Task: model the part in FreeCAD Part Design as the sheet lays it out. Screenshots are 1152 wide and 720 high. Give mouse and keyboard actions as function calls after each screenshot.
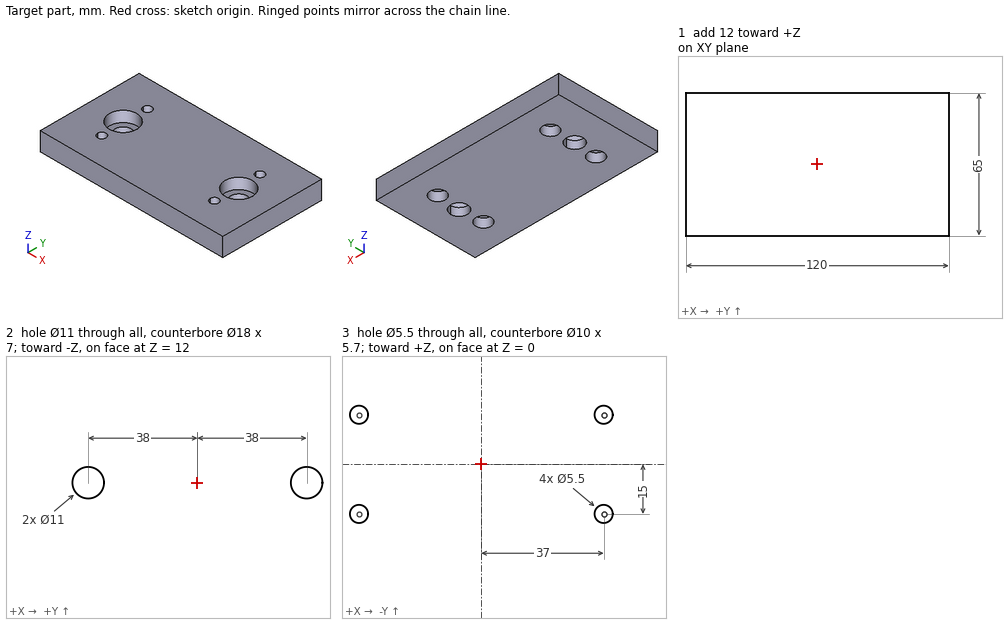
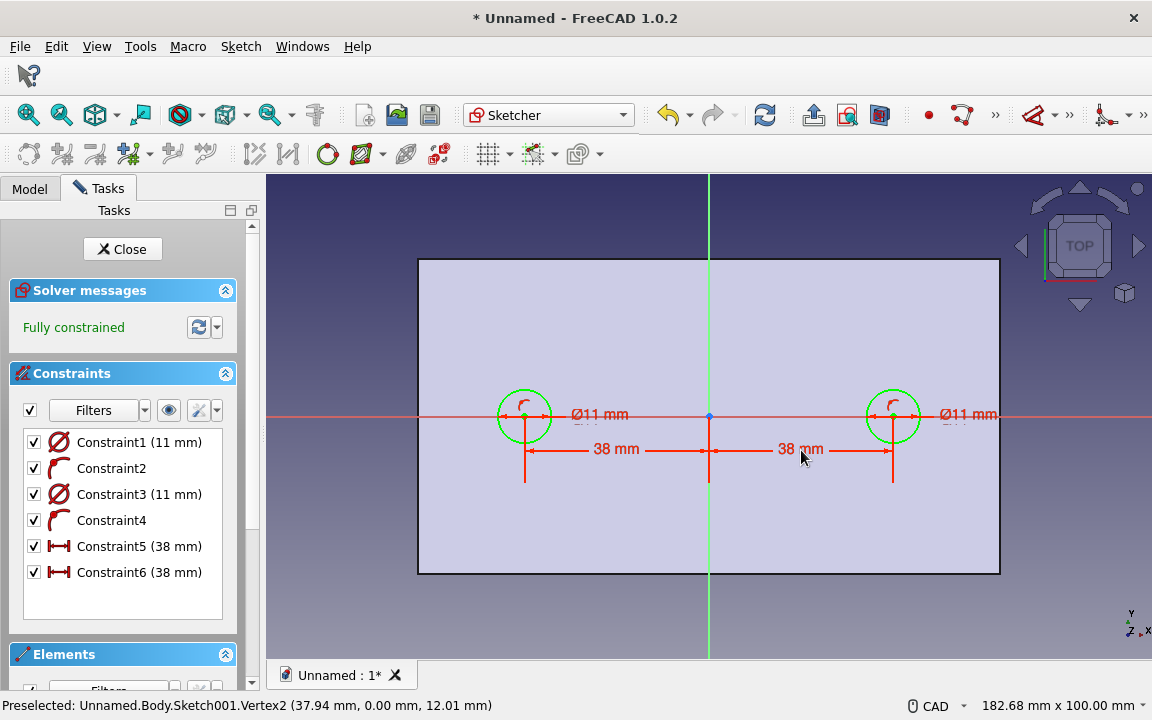
click(123, 249)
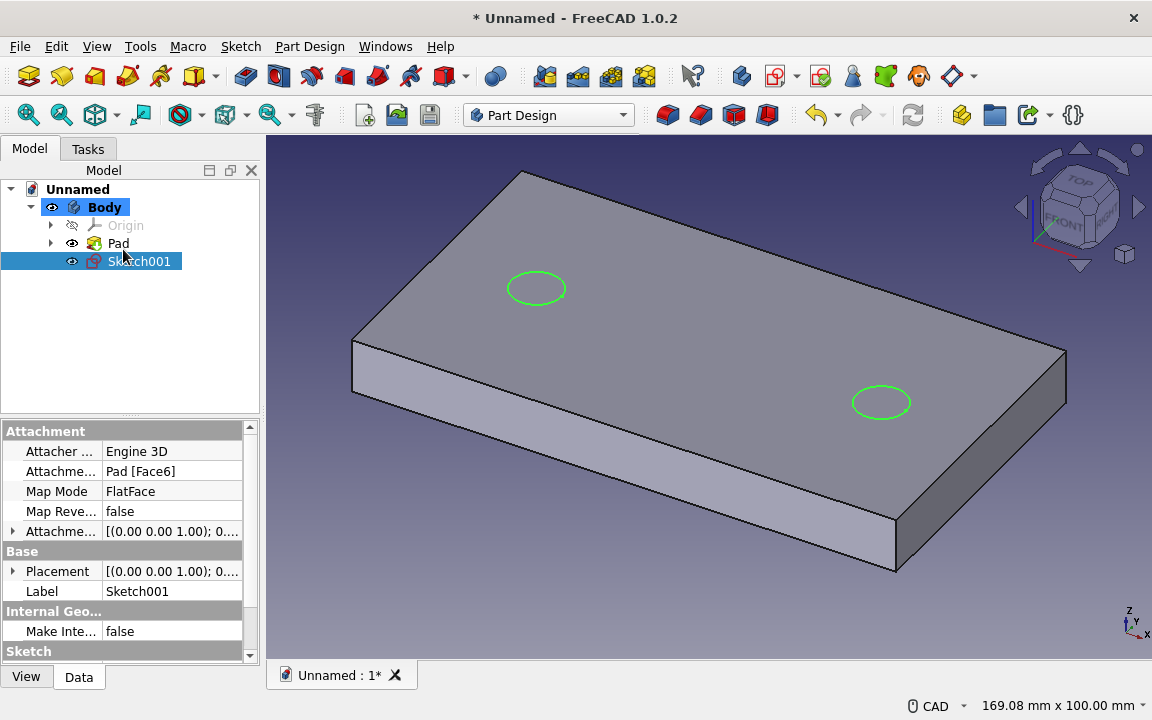
click(279, 76)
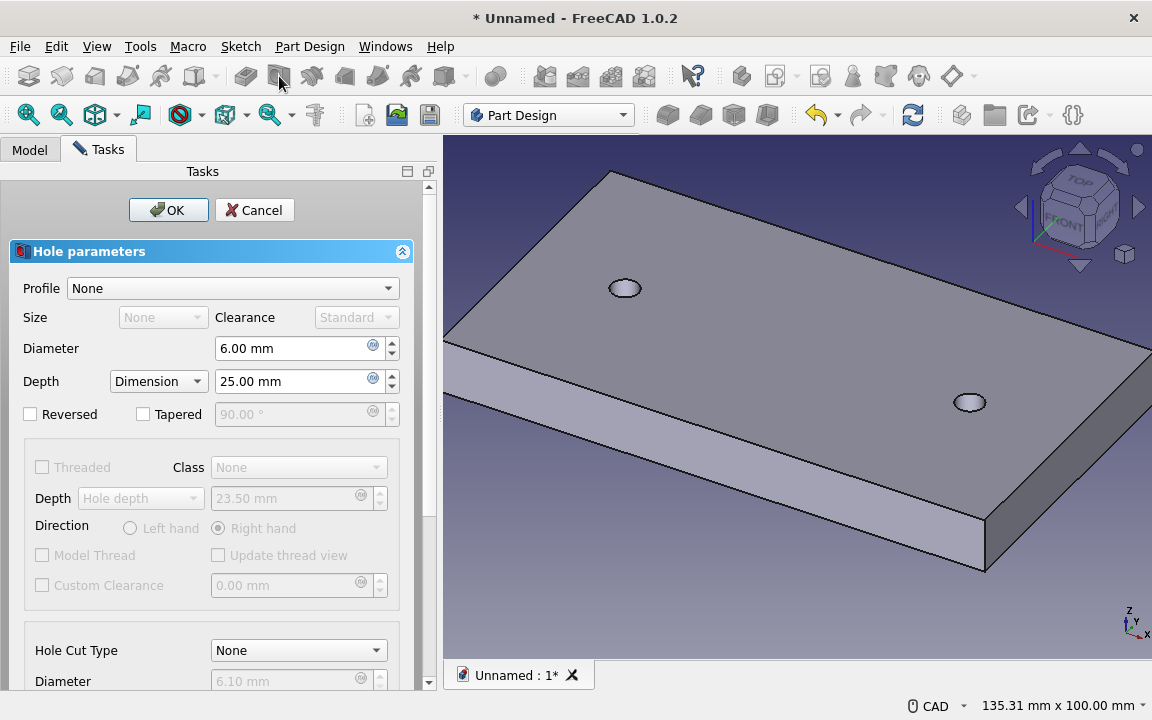
triple_click(300, 348)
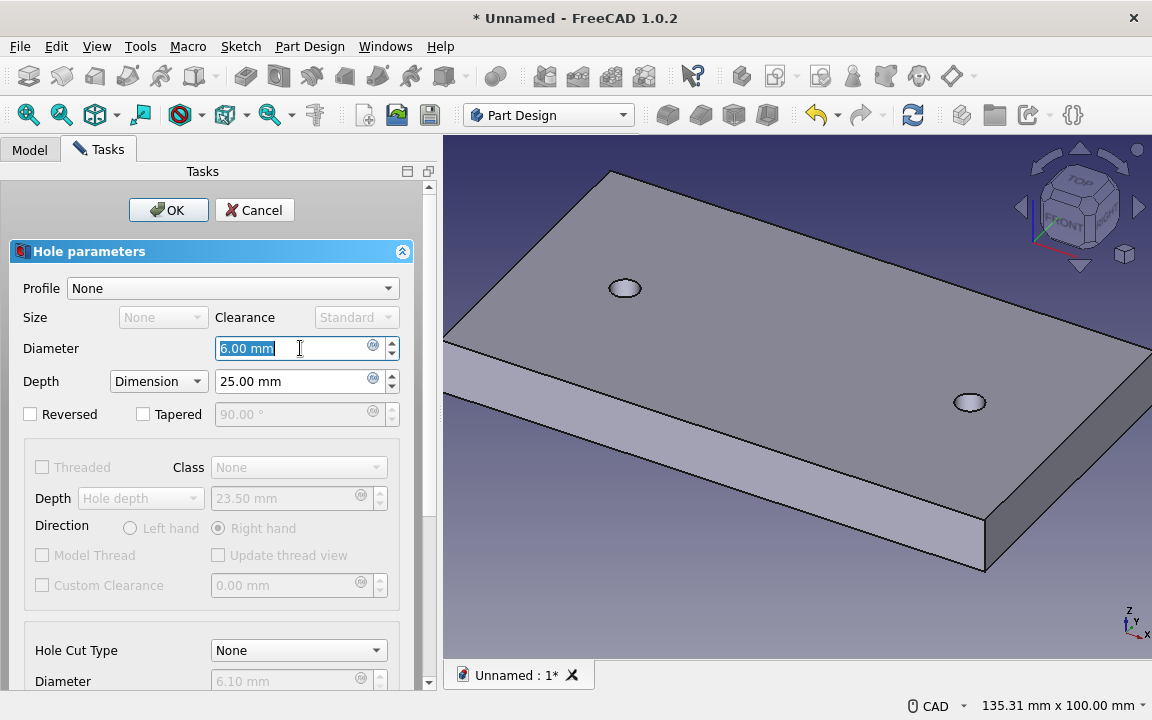
text(11)
key(Tab)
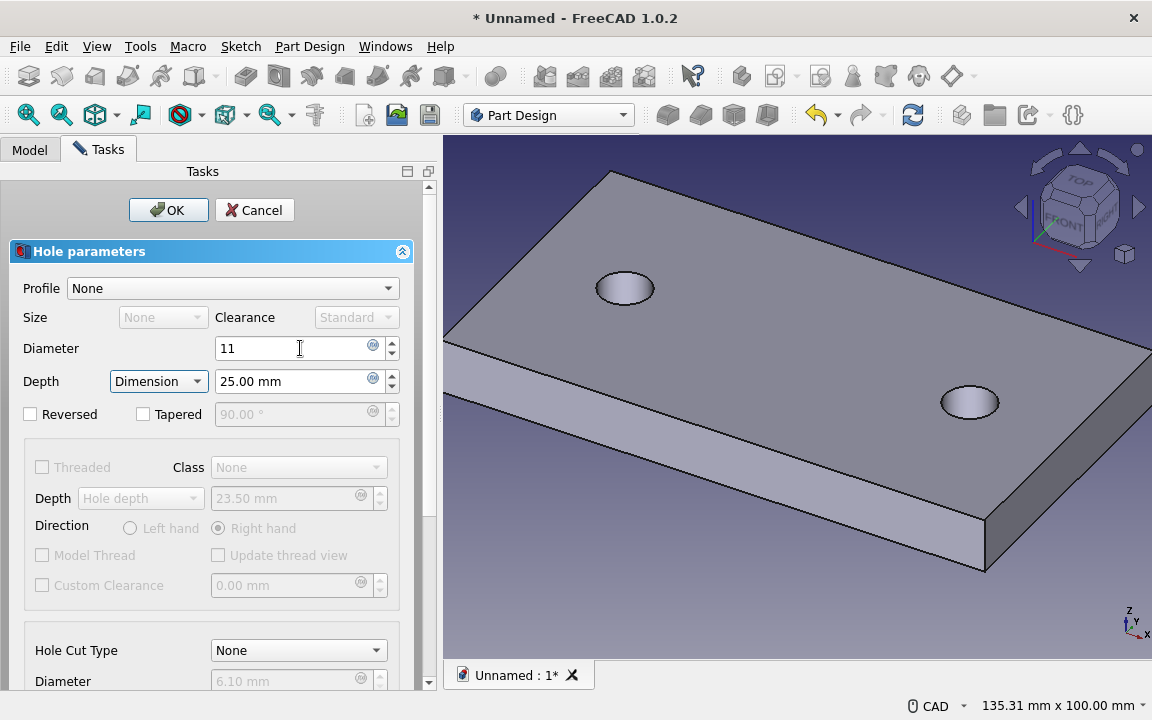
click(160, 382)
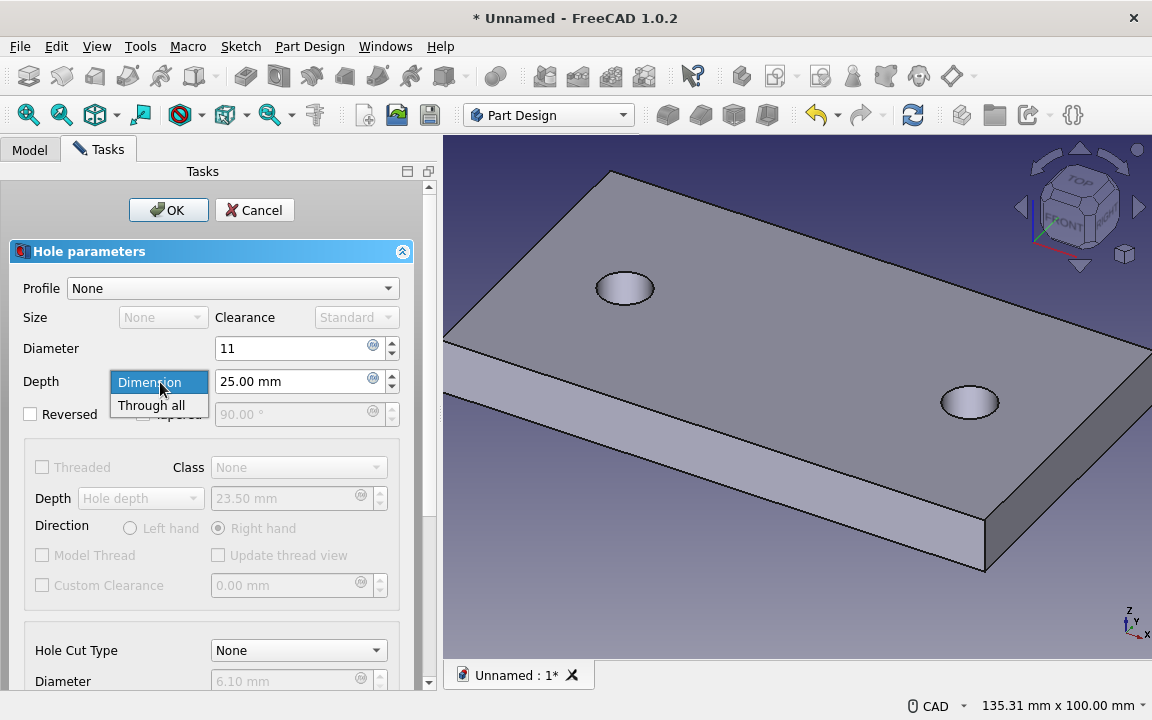
click(158, 406)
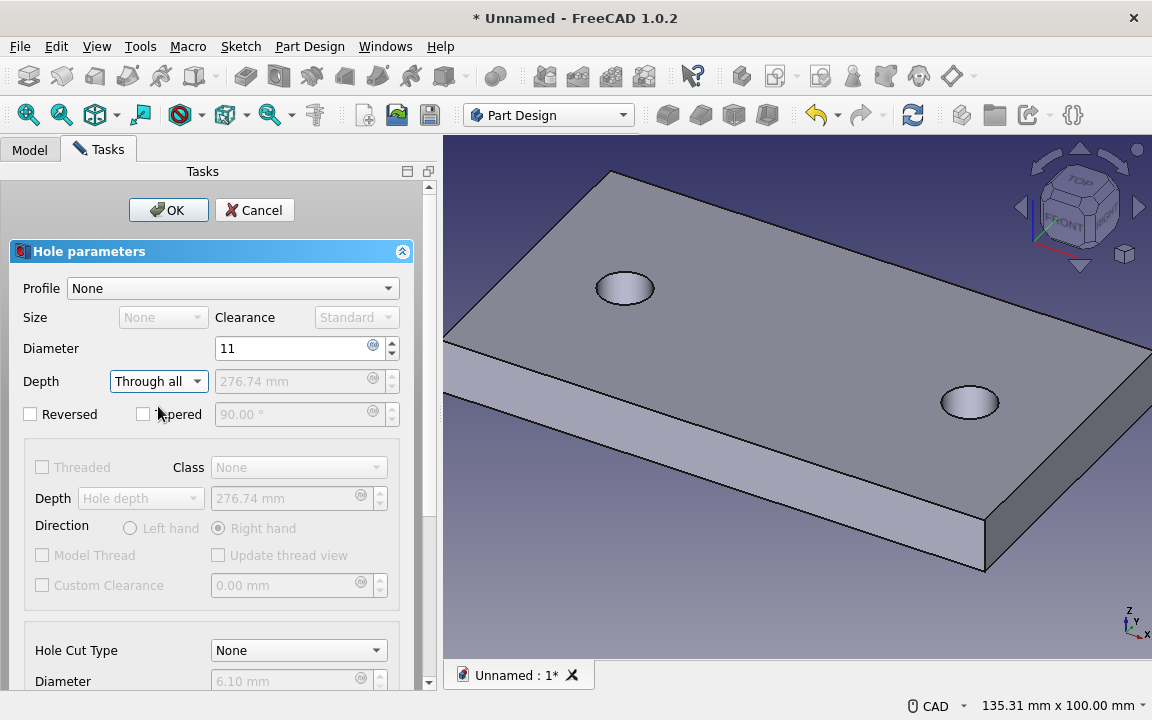
click(300, 650)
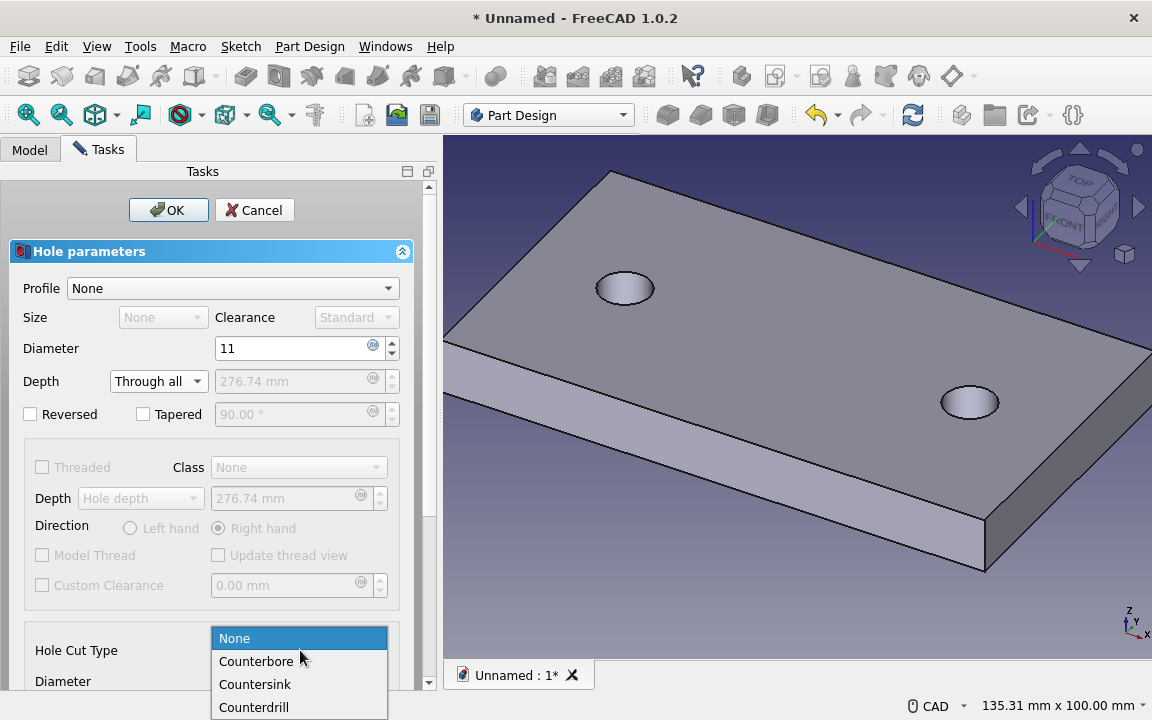
click(298, 662)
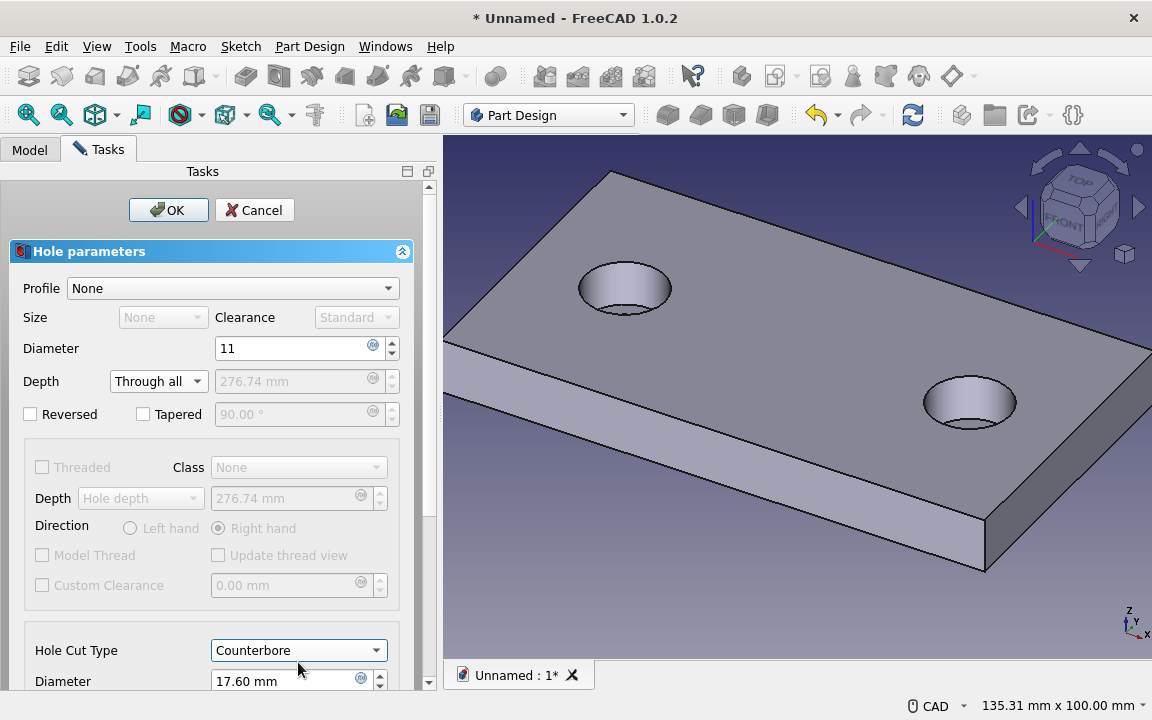
scroll(429, 436, down, 2)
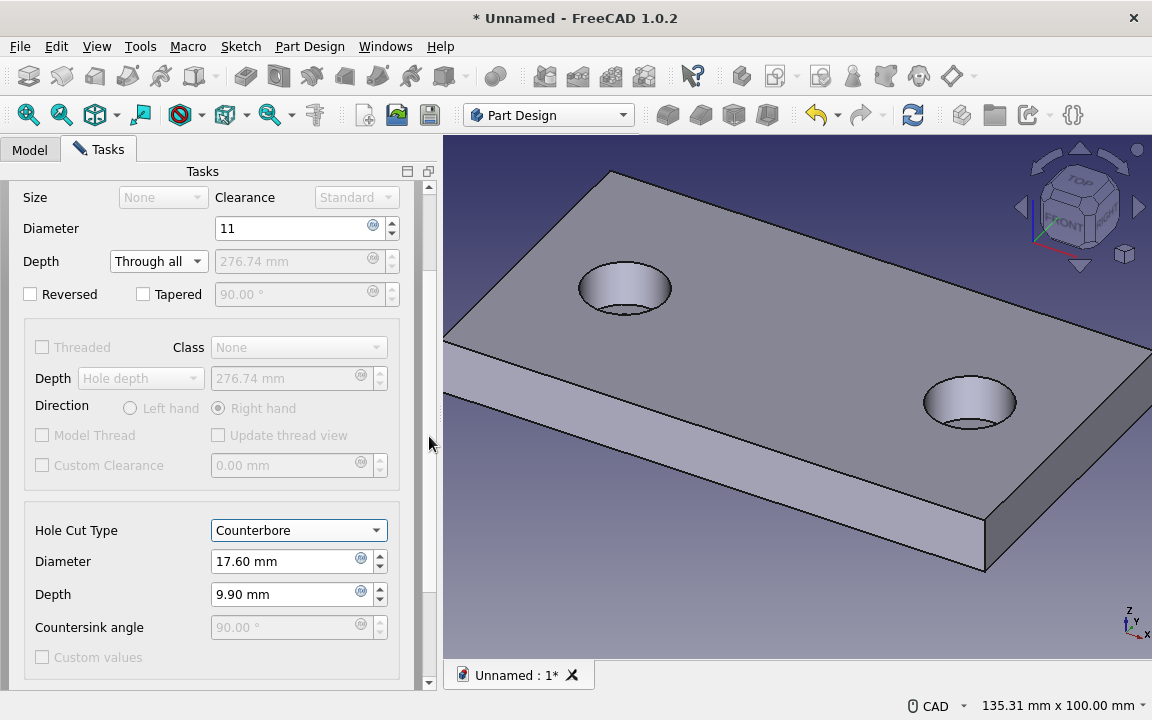
triple_click(292, 562)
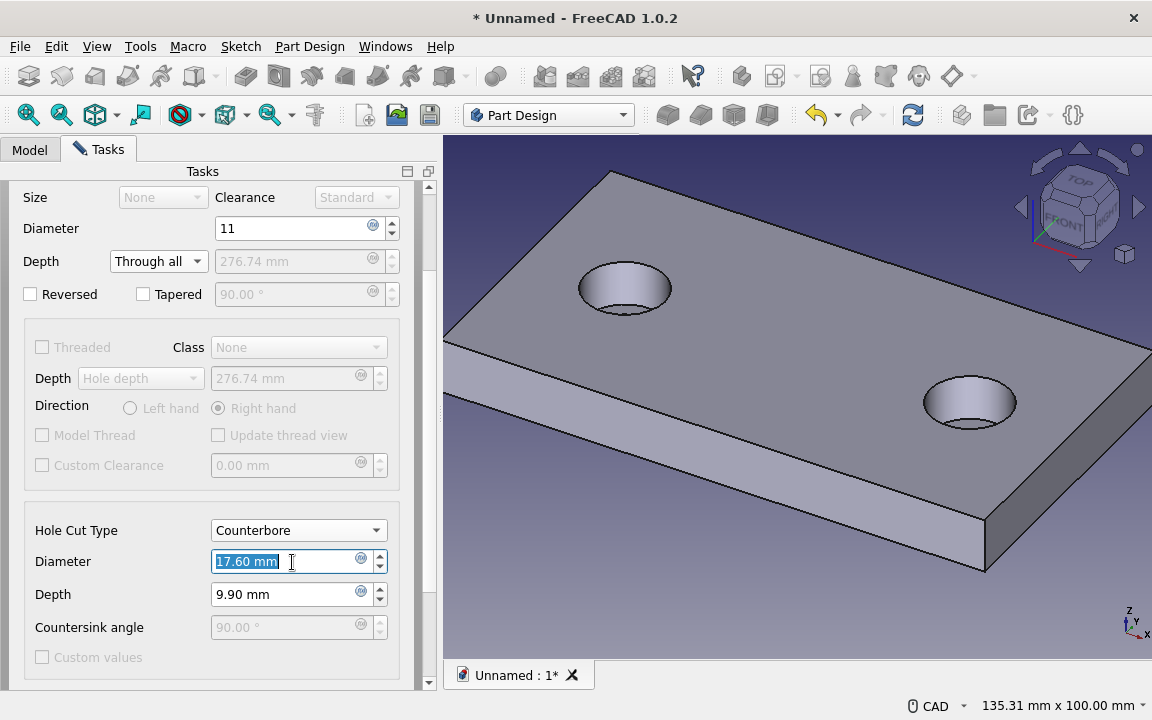
text(18)
key(Tab)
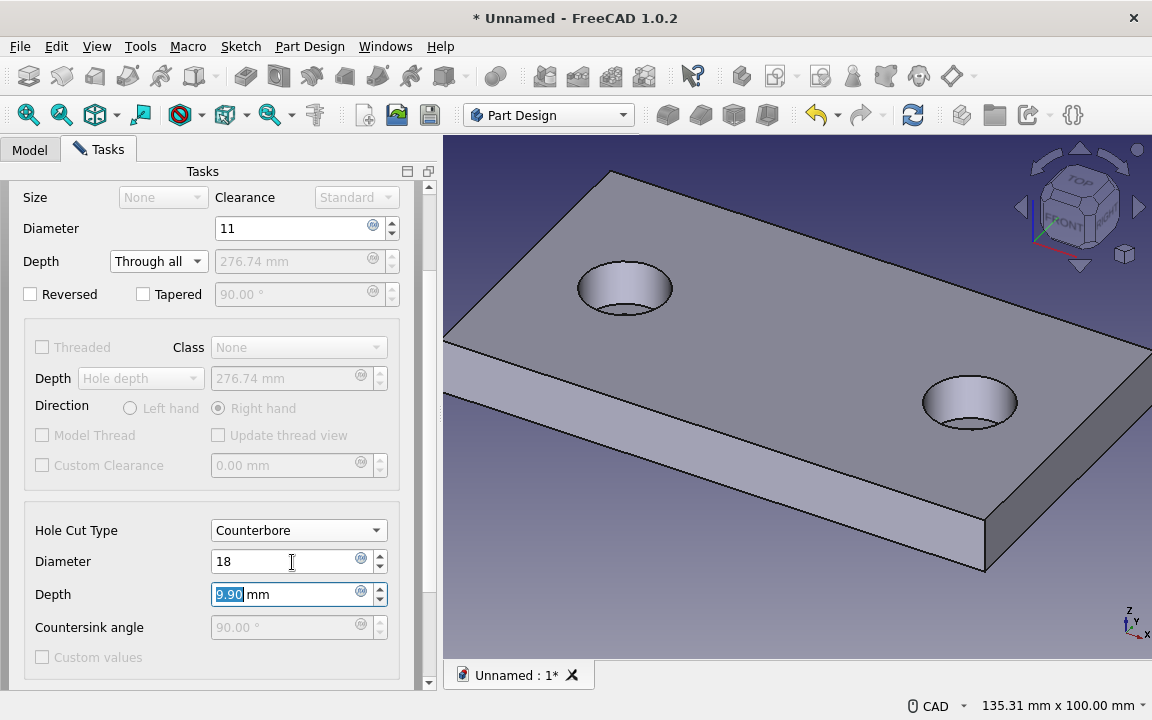
text(7)
key(Tab)